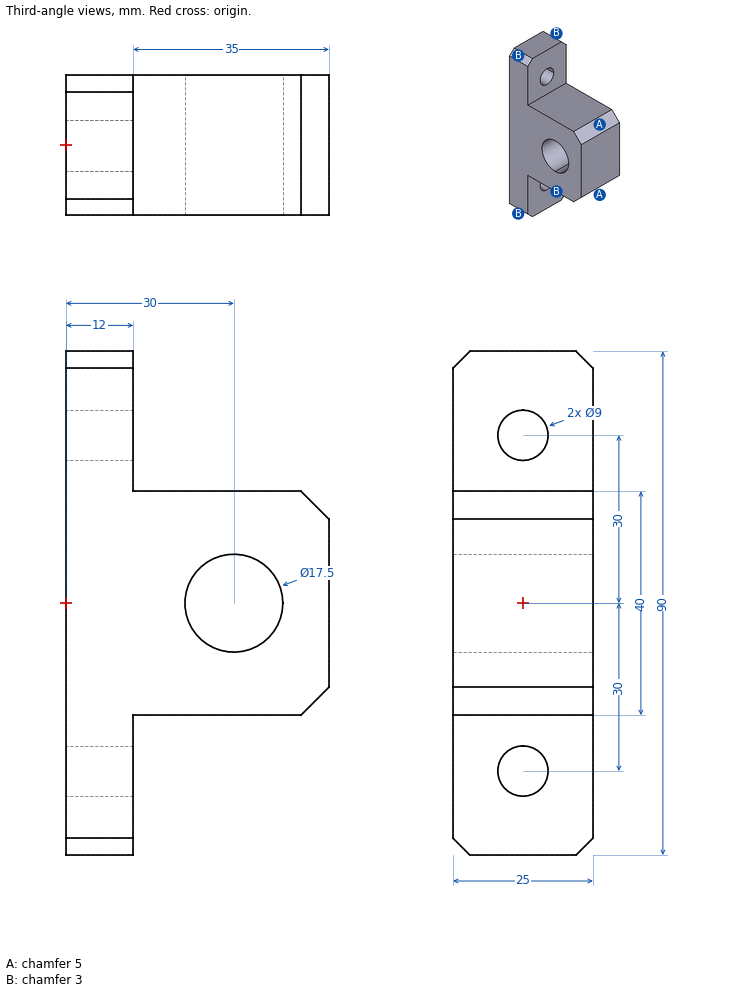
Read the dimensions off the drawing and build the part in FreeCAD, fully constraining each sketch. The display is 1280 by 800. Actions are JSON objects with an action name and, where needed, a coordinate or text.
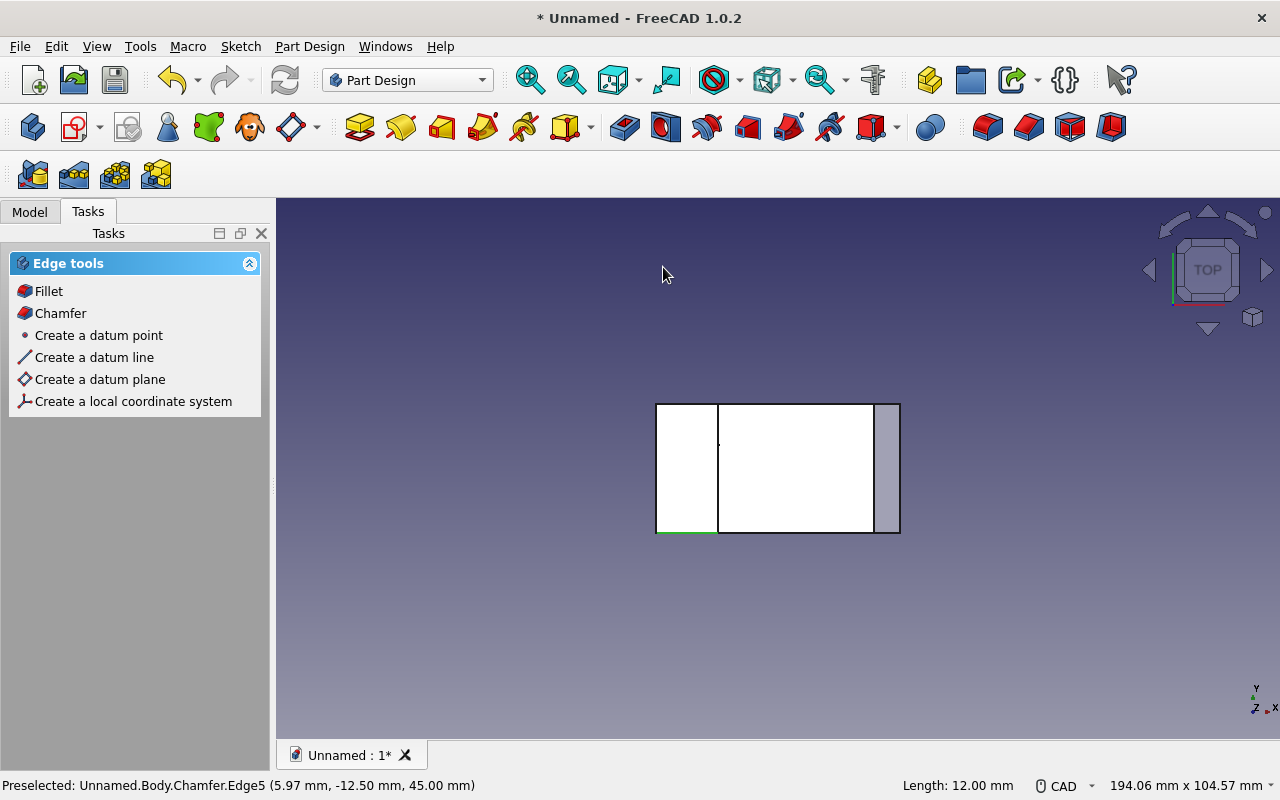
{"action": "left_click", "coordinate": [531, 80]}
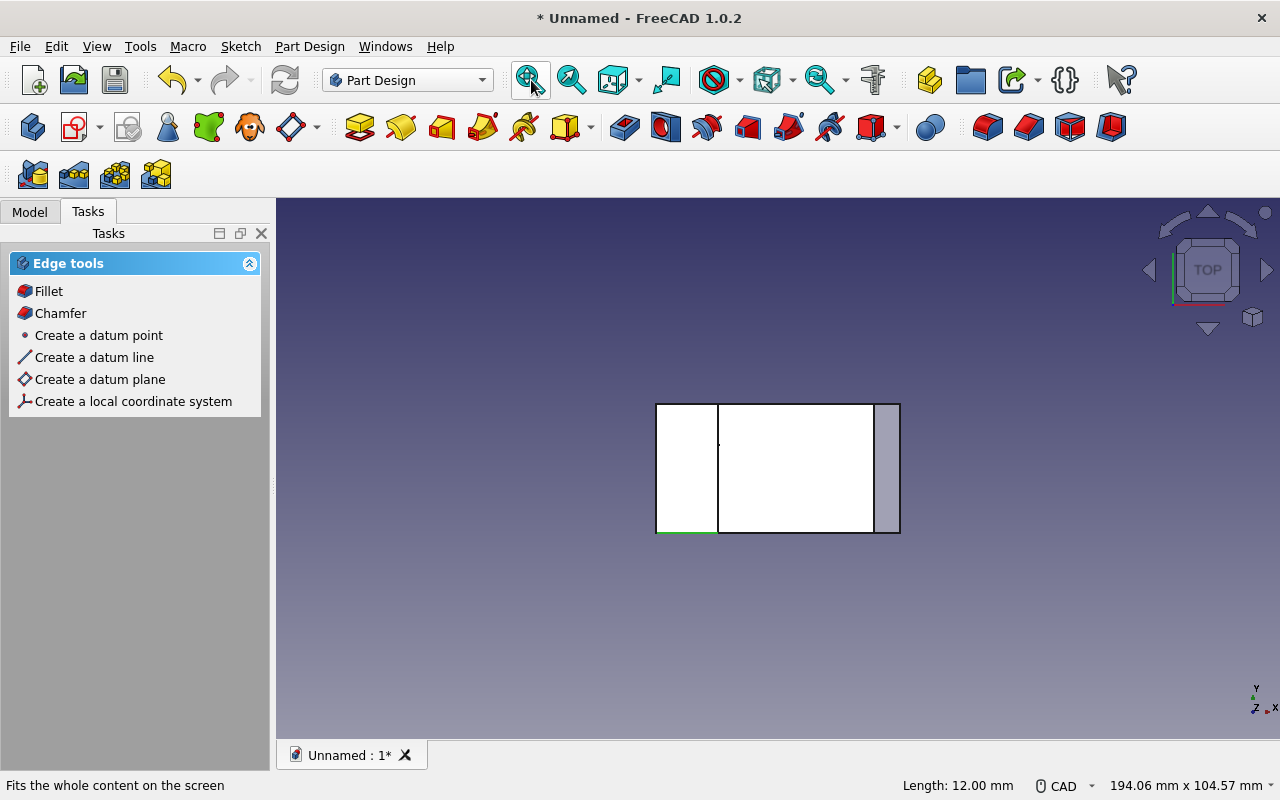
{"action": "left_click", "coordinate": [687, 403], "text": "ctrl"}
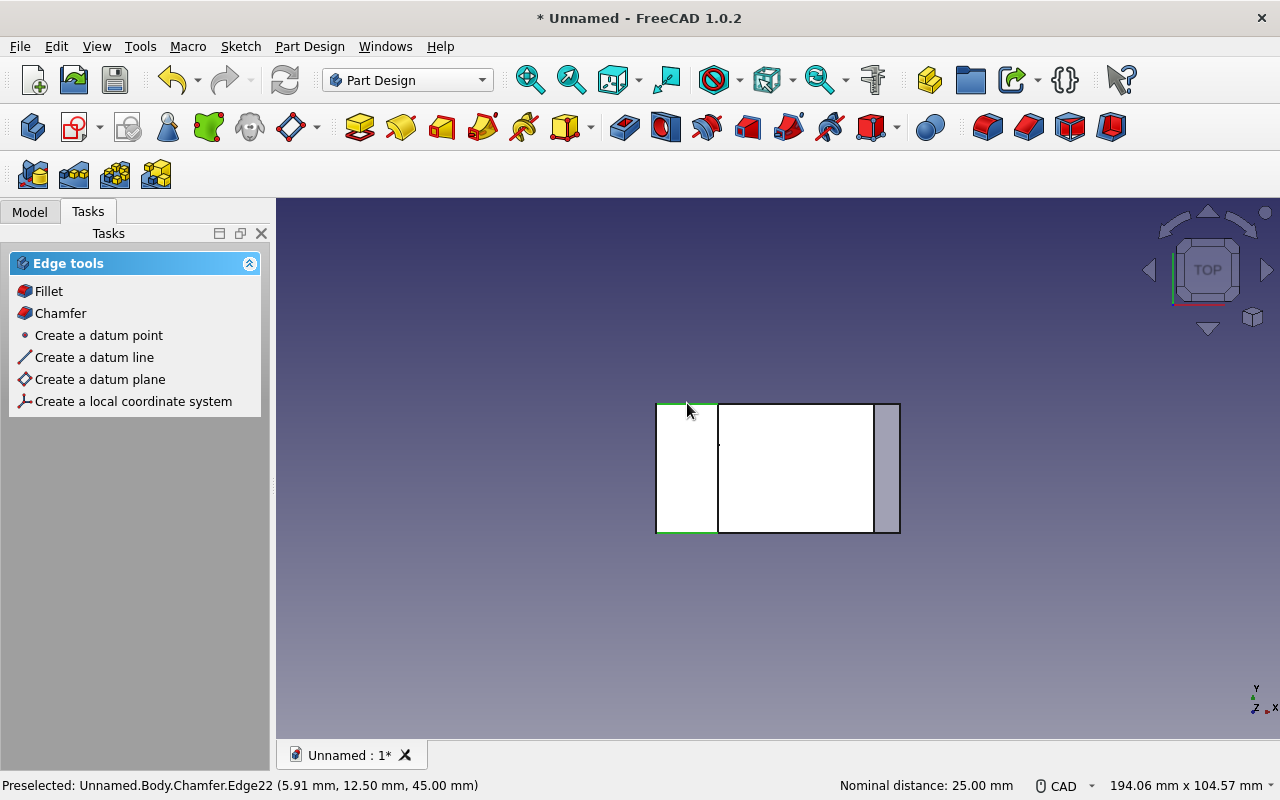
{"action": "key", "text": "1"}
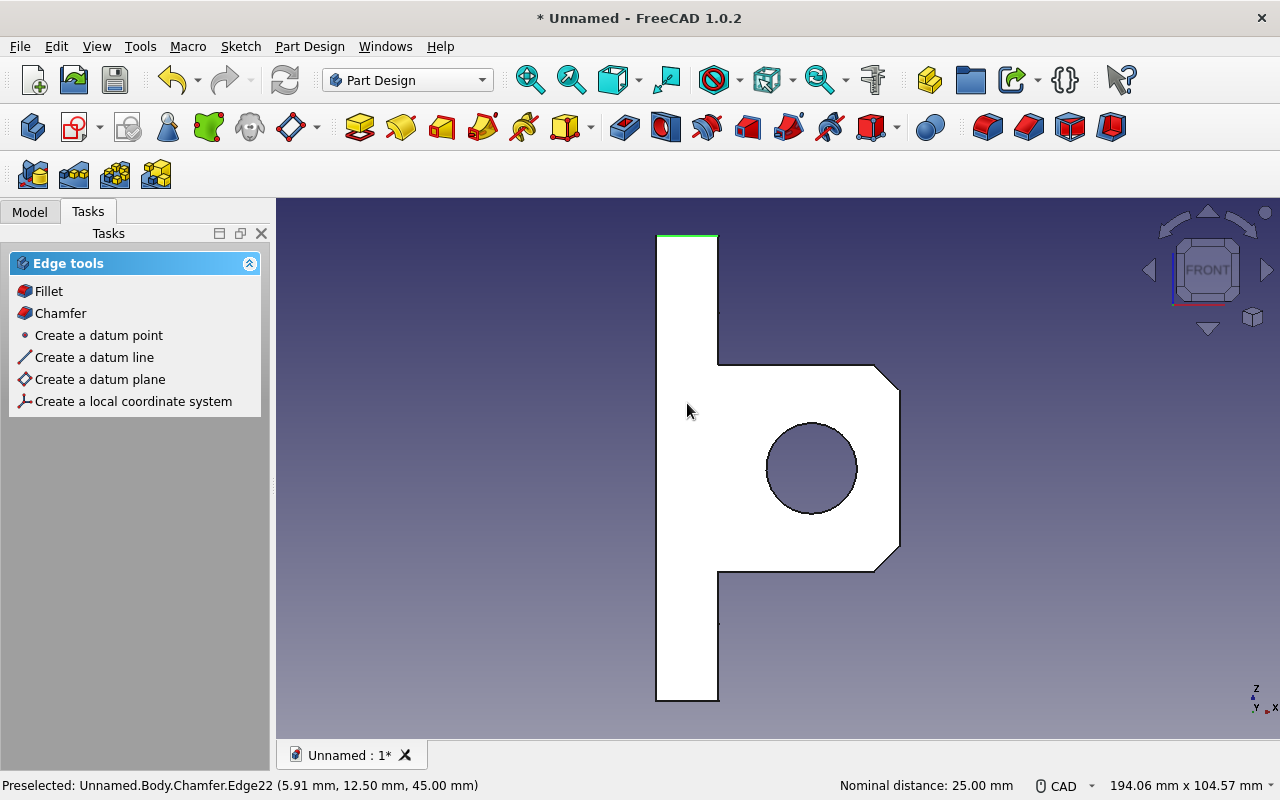
{"action": "left_click", "coordinate": [687, 700], "text": "ctrl"}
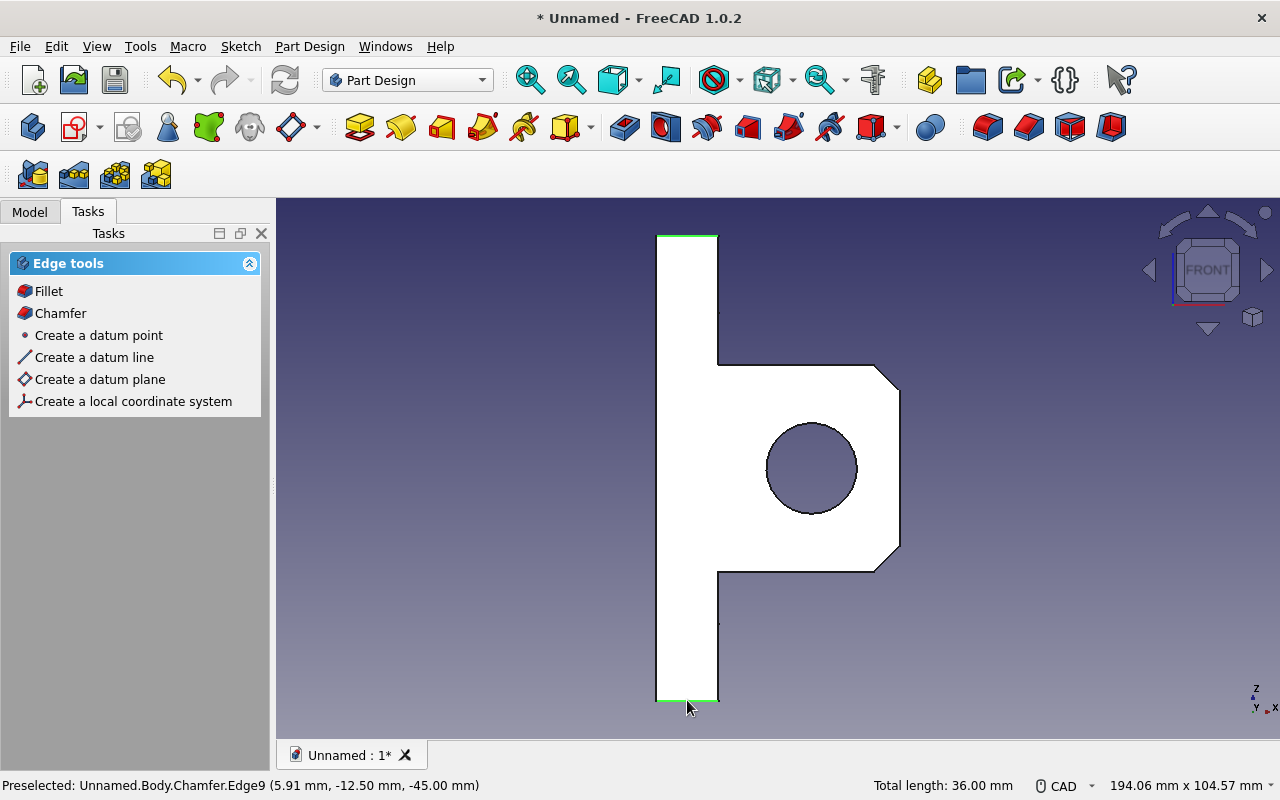
{"action": "key", "text": "3"}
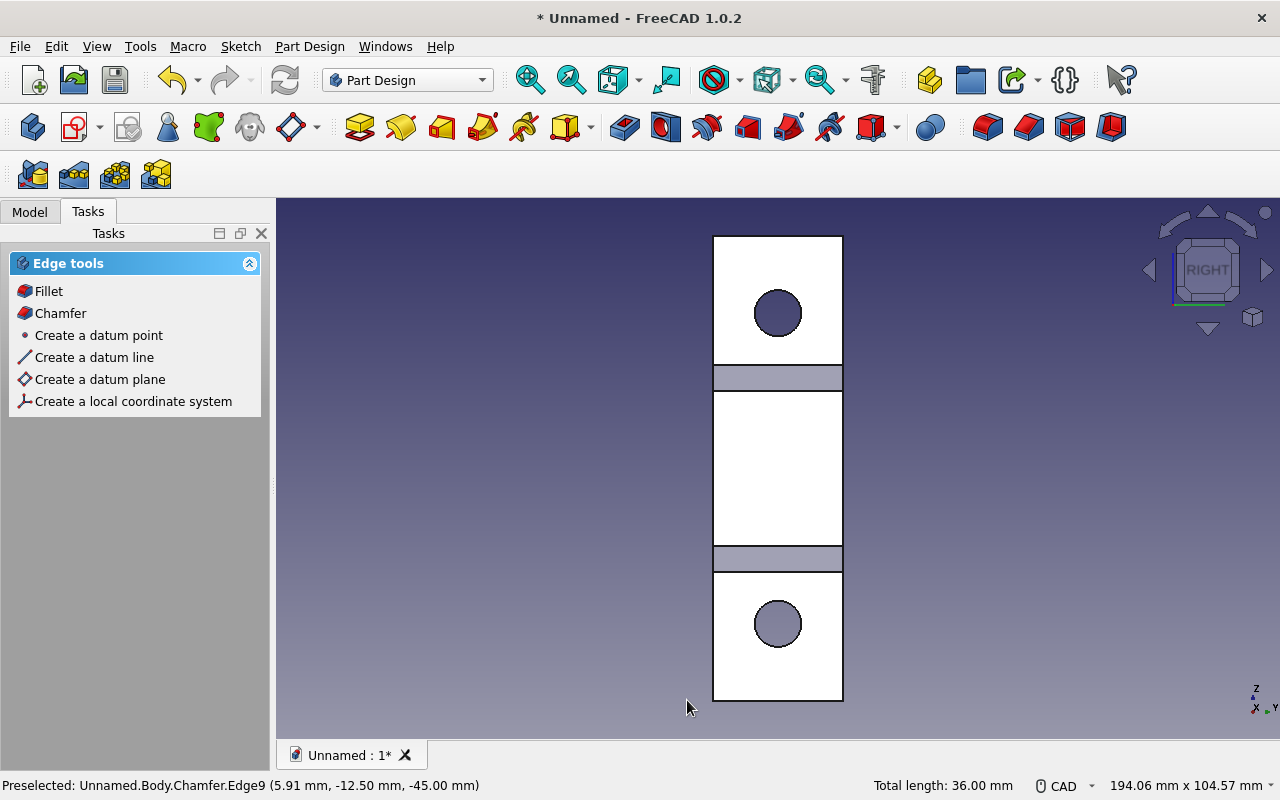
{"action": "key", "text": "5"}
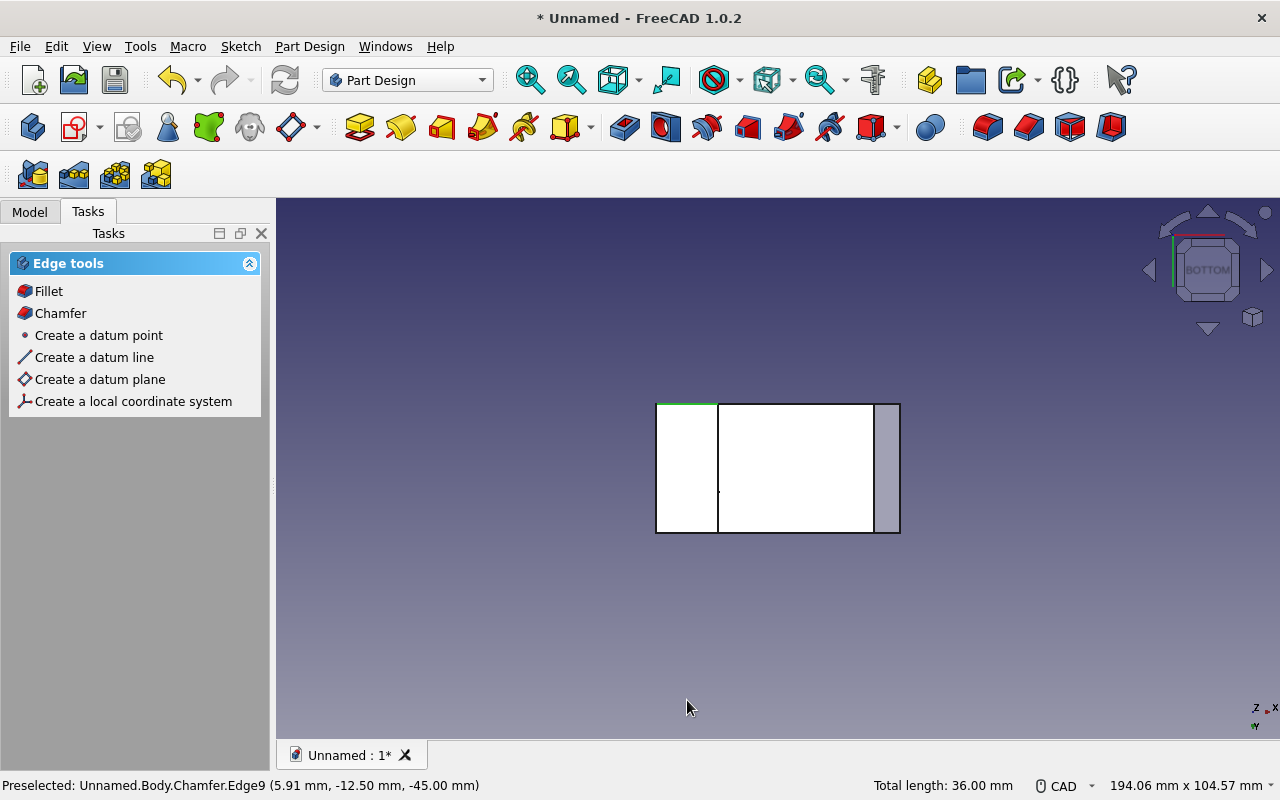
{"action": "key", "text": "v f"}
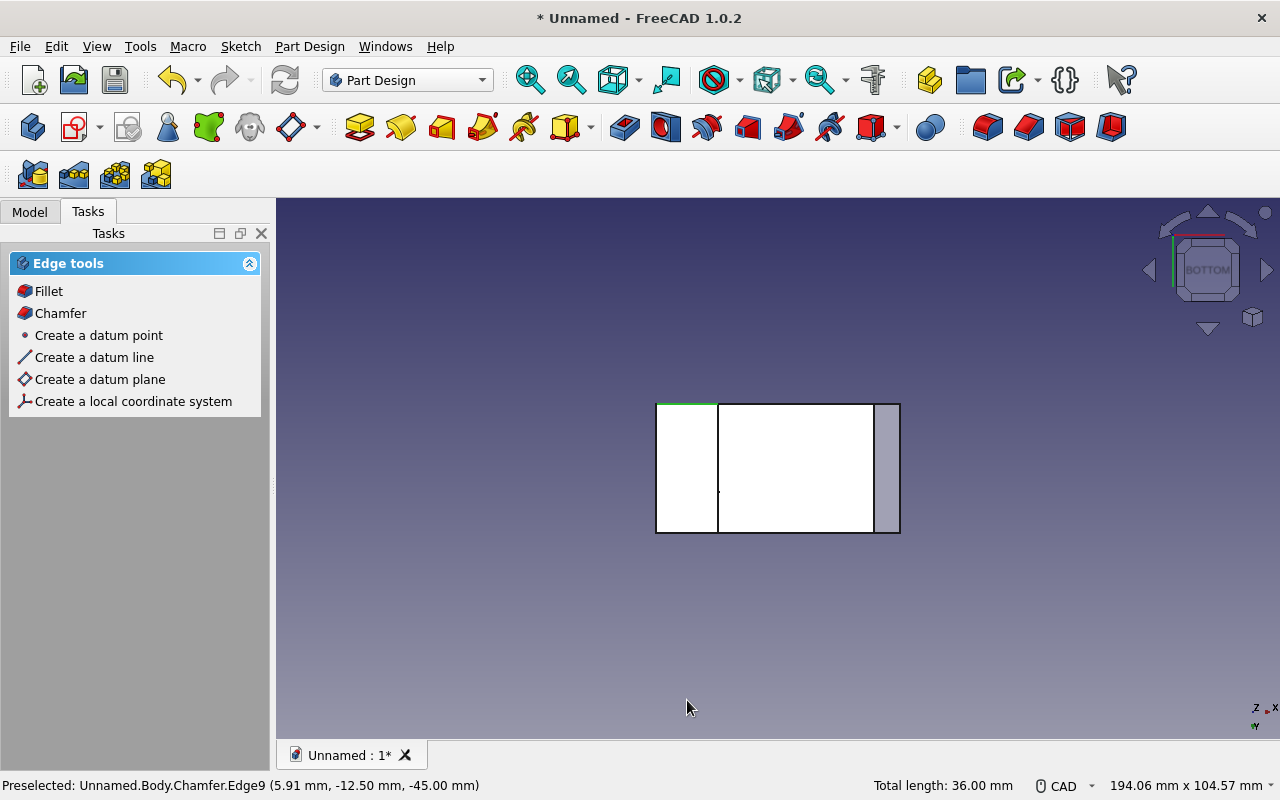
{"action": "left_click", "coordinate": [687, 532], "text": "ctrl"}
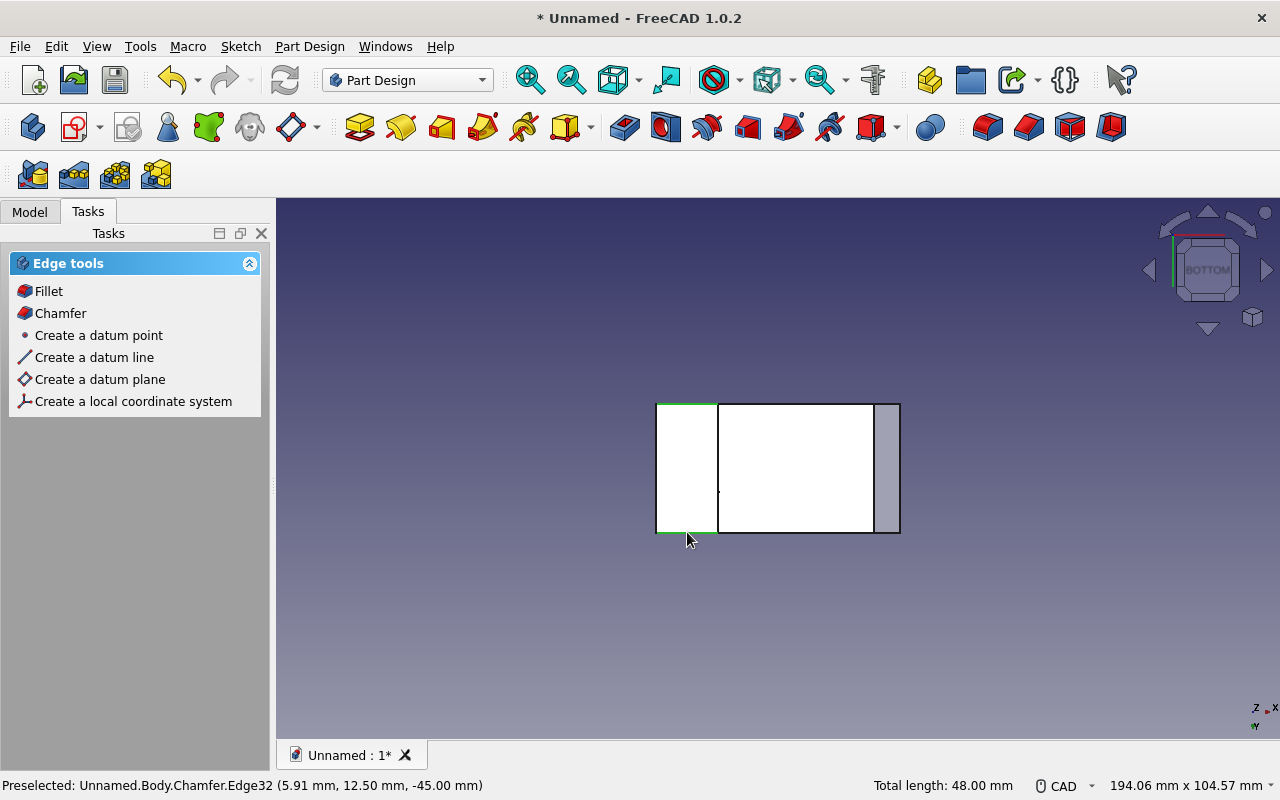
{"action": "left_click", "coordinate": [1029, 128]}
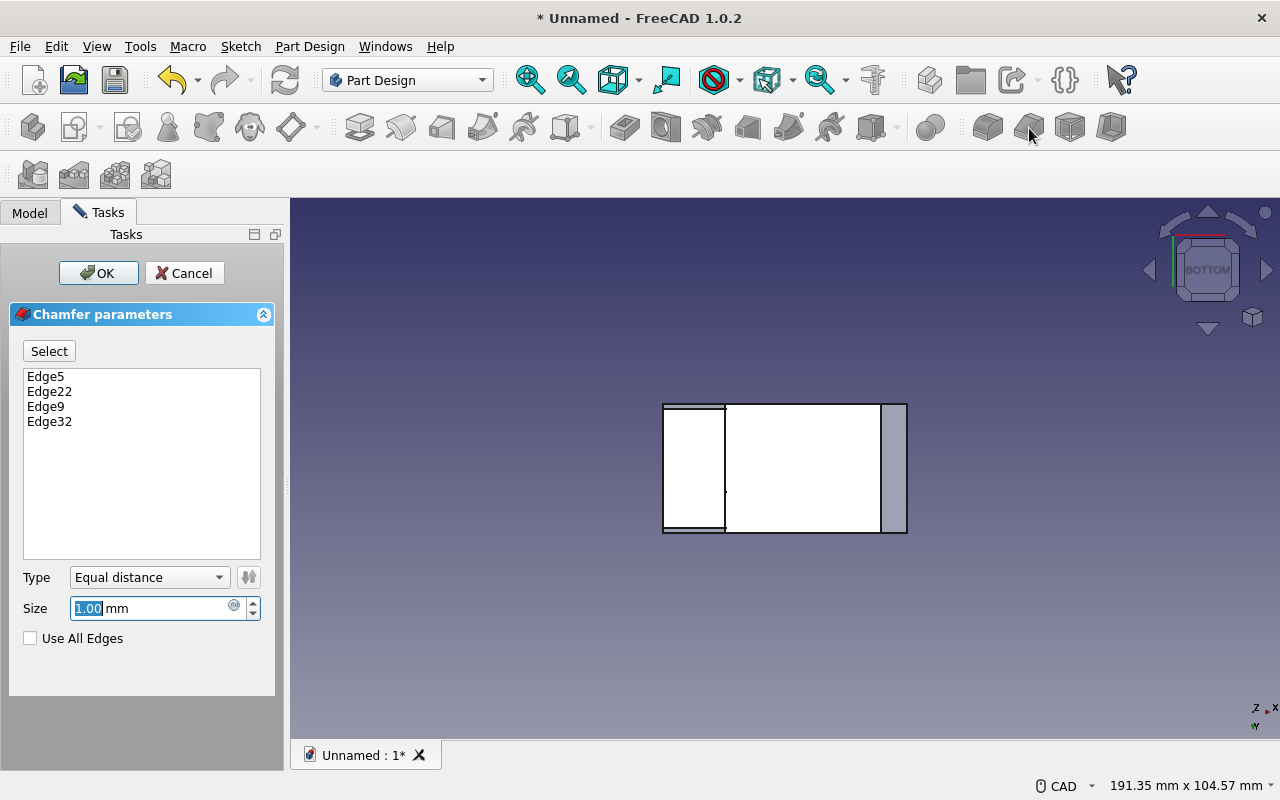
{"action": "type", "text": "3"}
{"action": "key", "text": "Tab"}